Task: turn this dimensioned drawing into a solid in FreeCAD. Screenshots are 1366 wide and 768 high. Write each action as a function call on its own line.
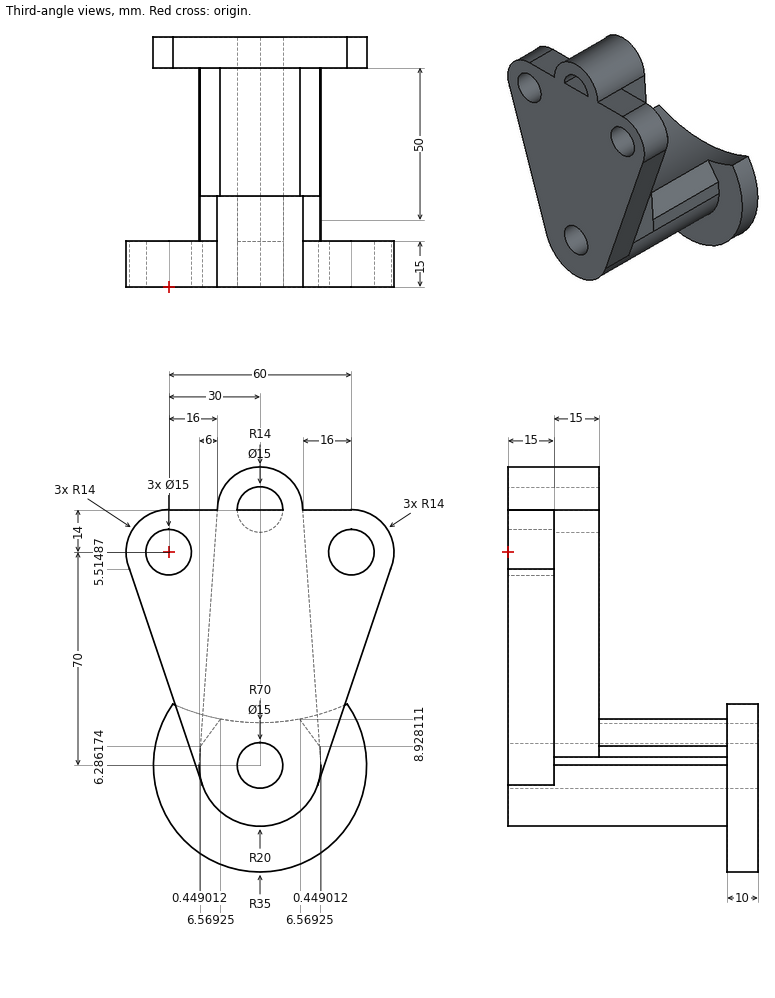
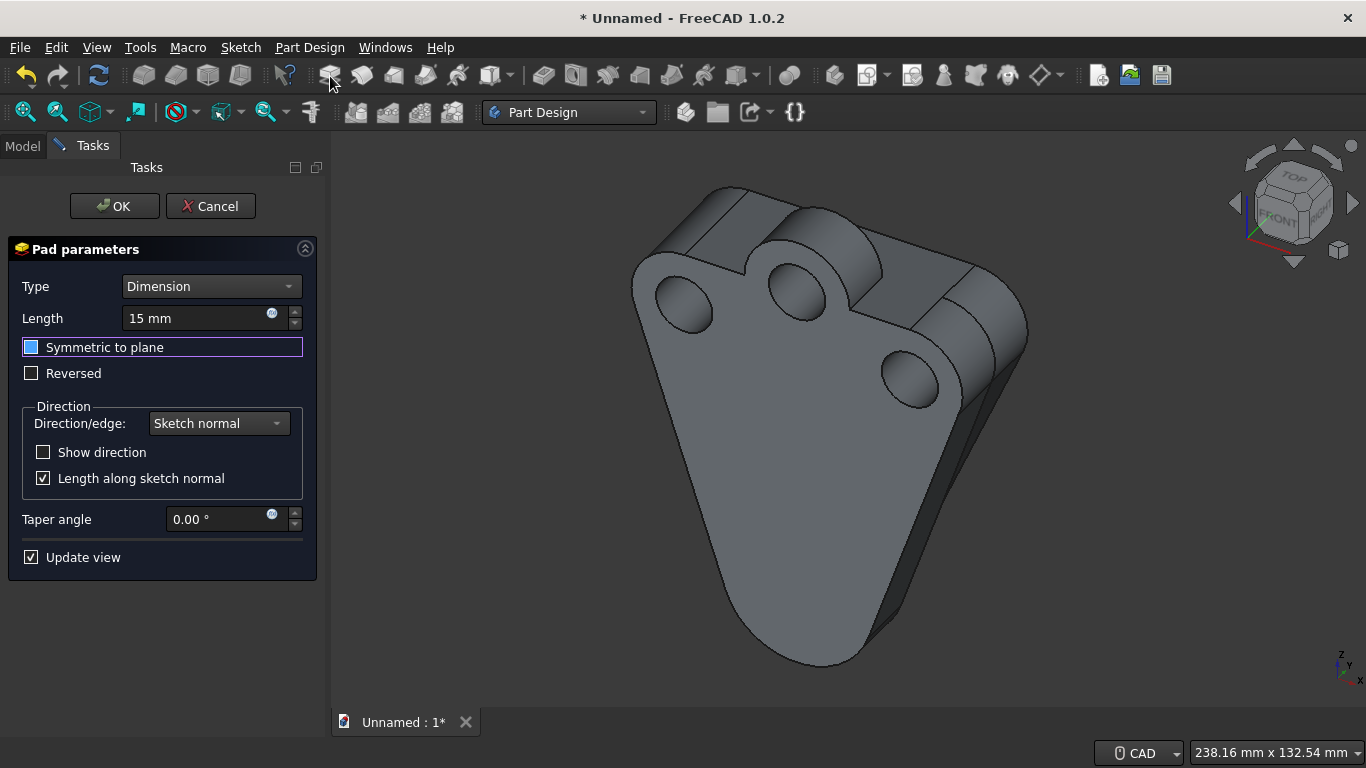
click(30, 373)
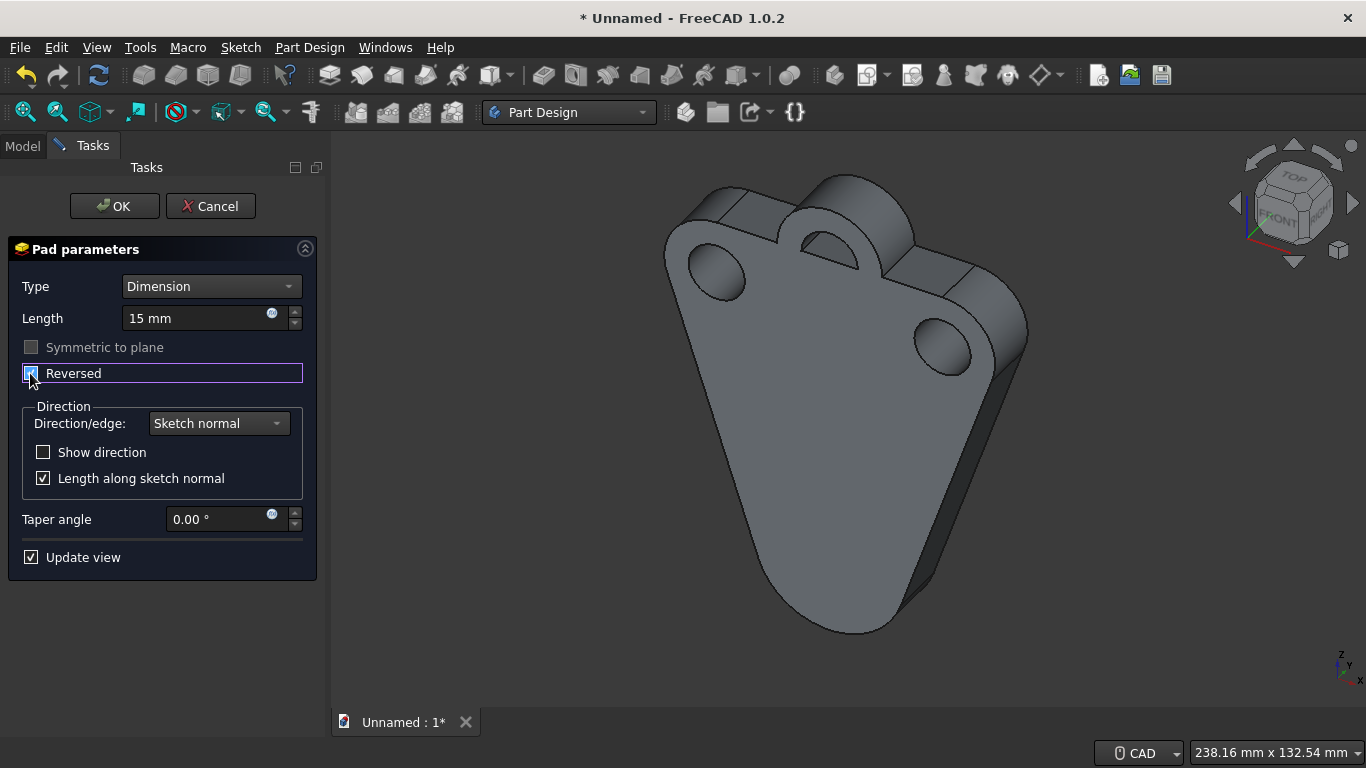
click(115, 206)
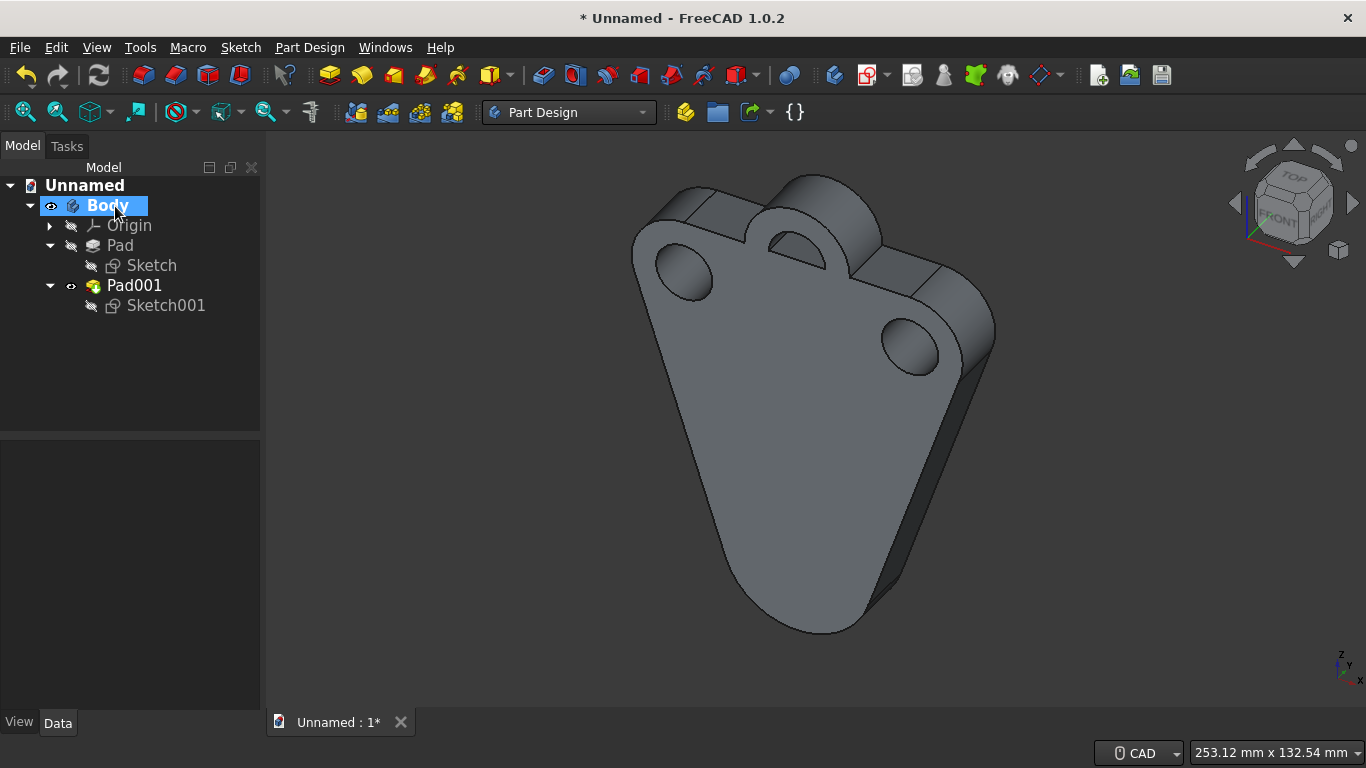
click(26, 112)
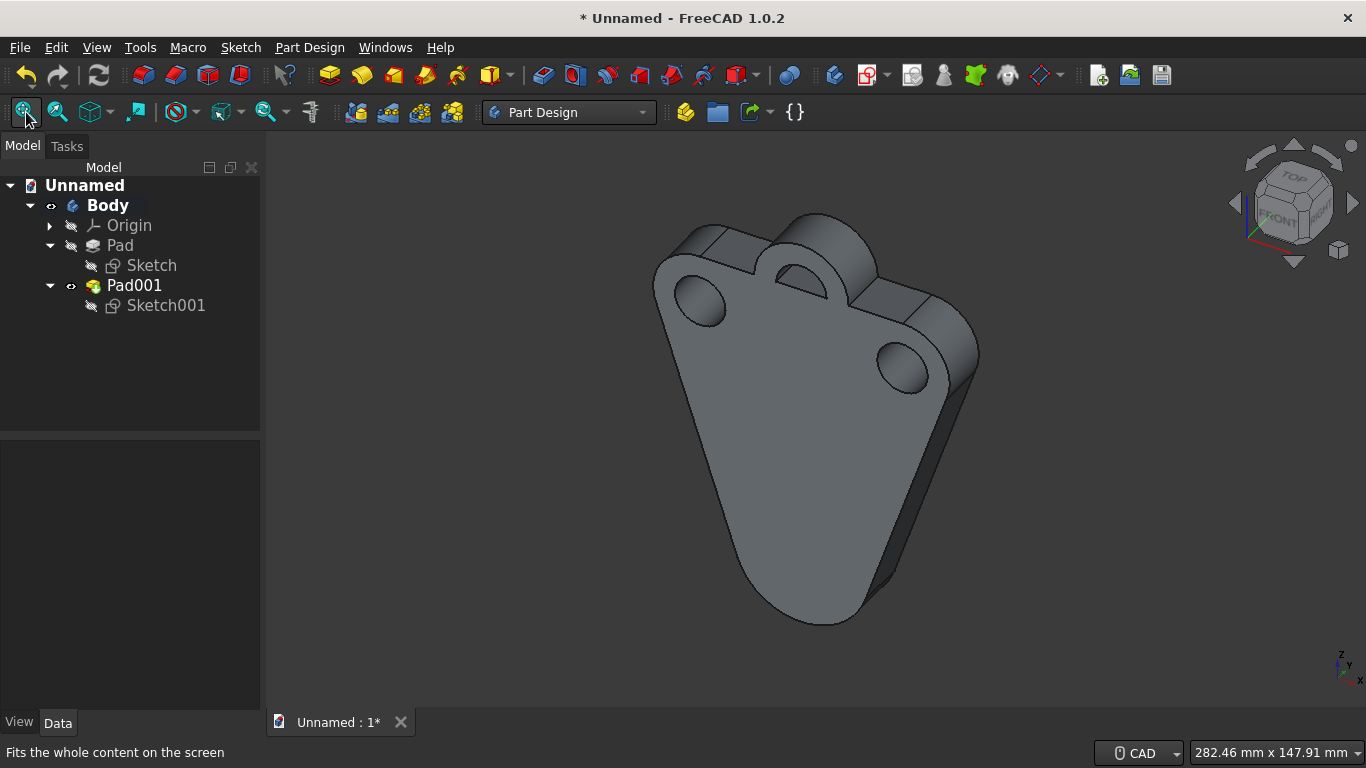
key(4)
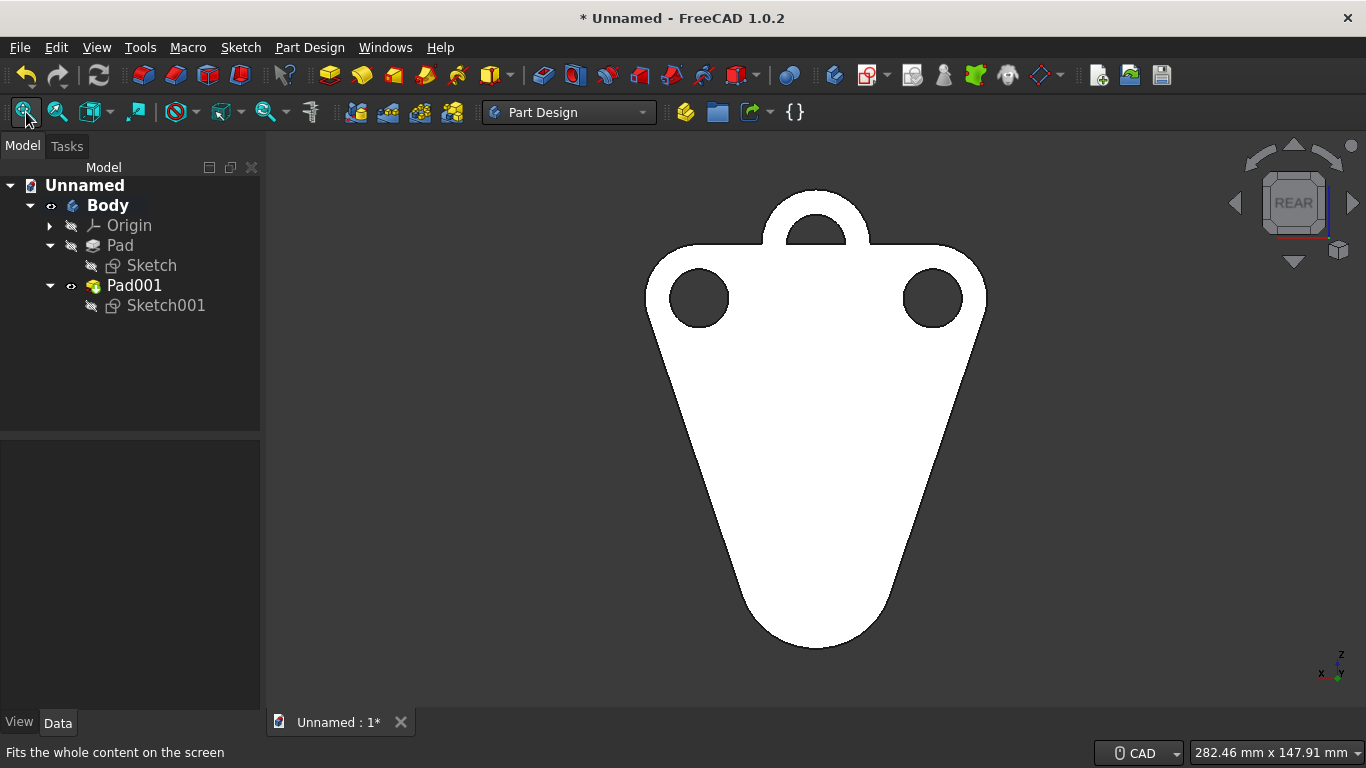
click(816, 418)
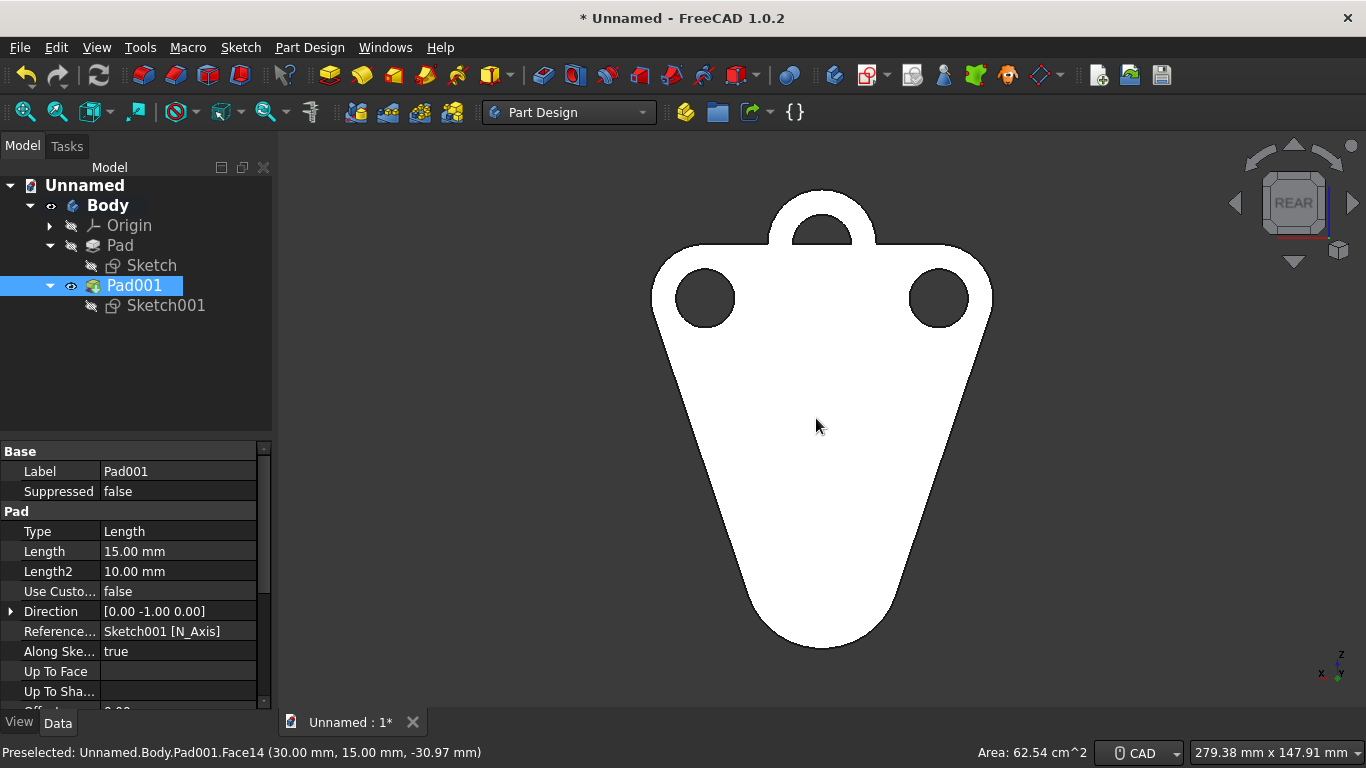
click(868, 76)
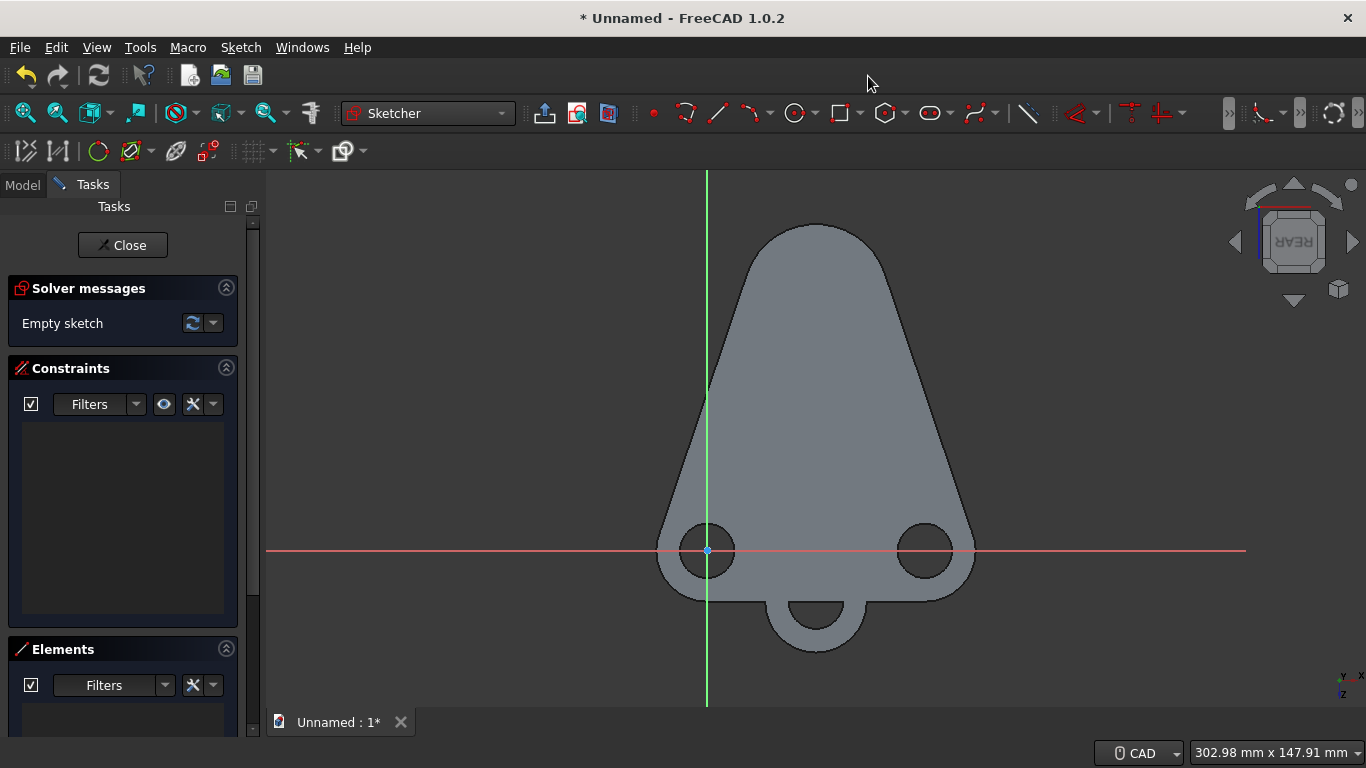
click(718, 114)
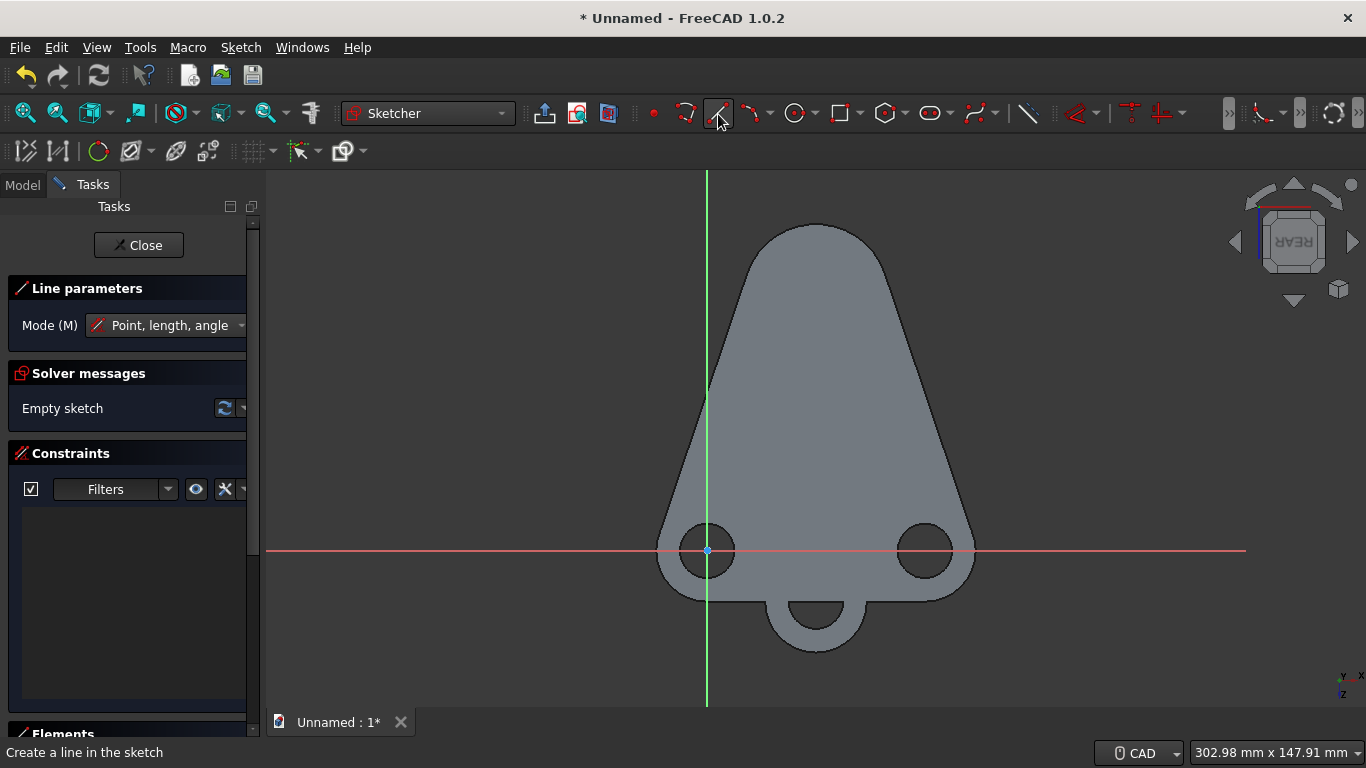
click(743, 297)
click(765, 602)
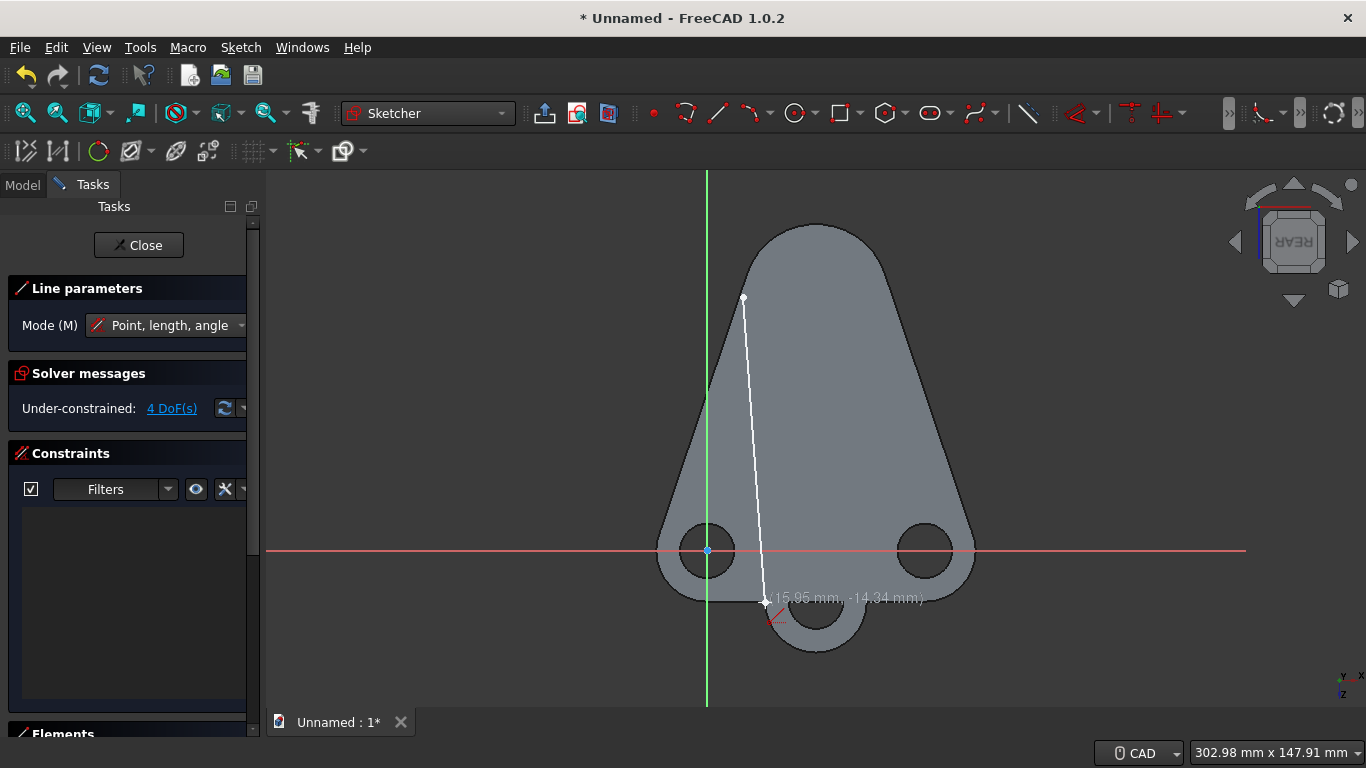
click(867, 602)
click(889, 297)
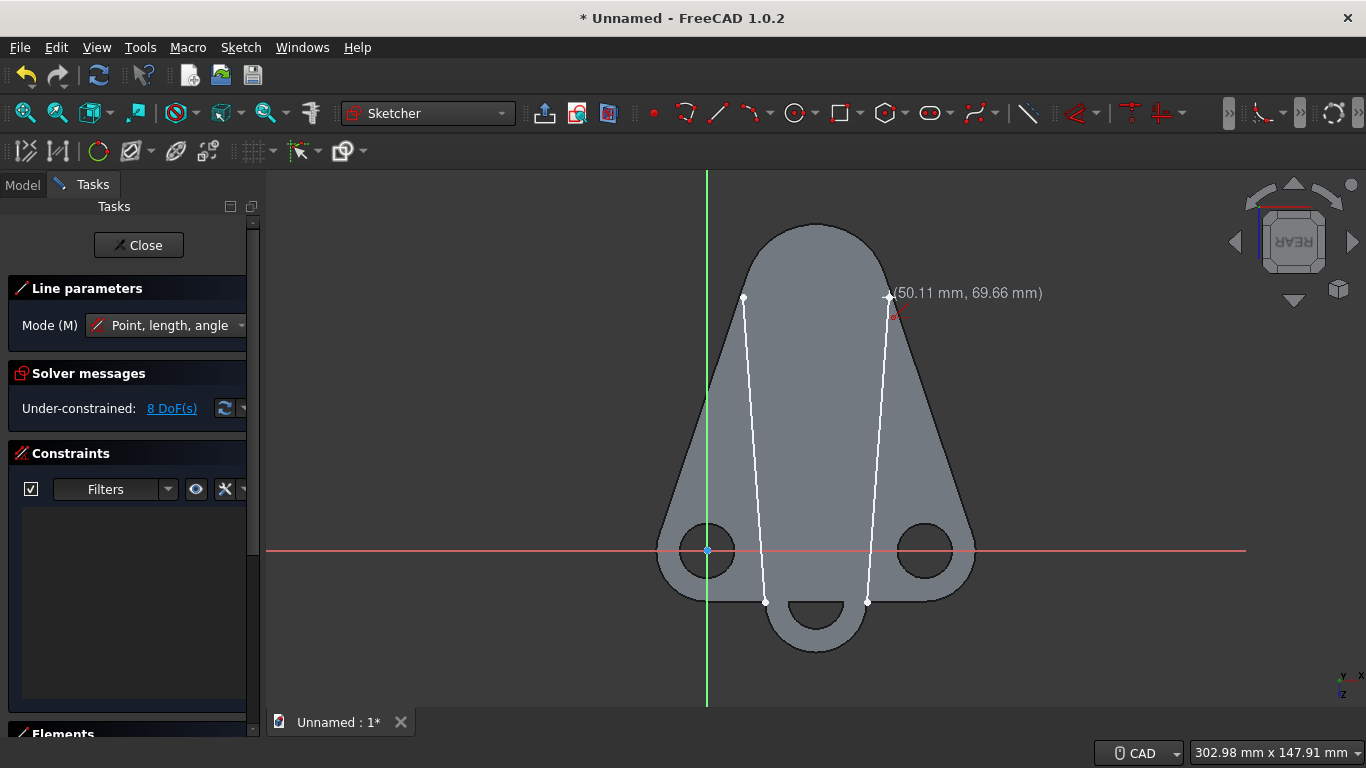
click(750, 114)